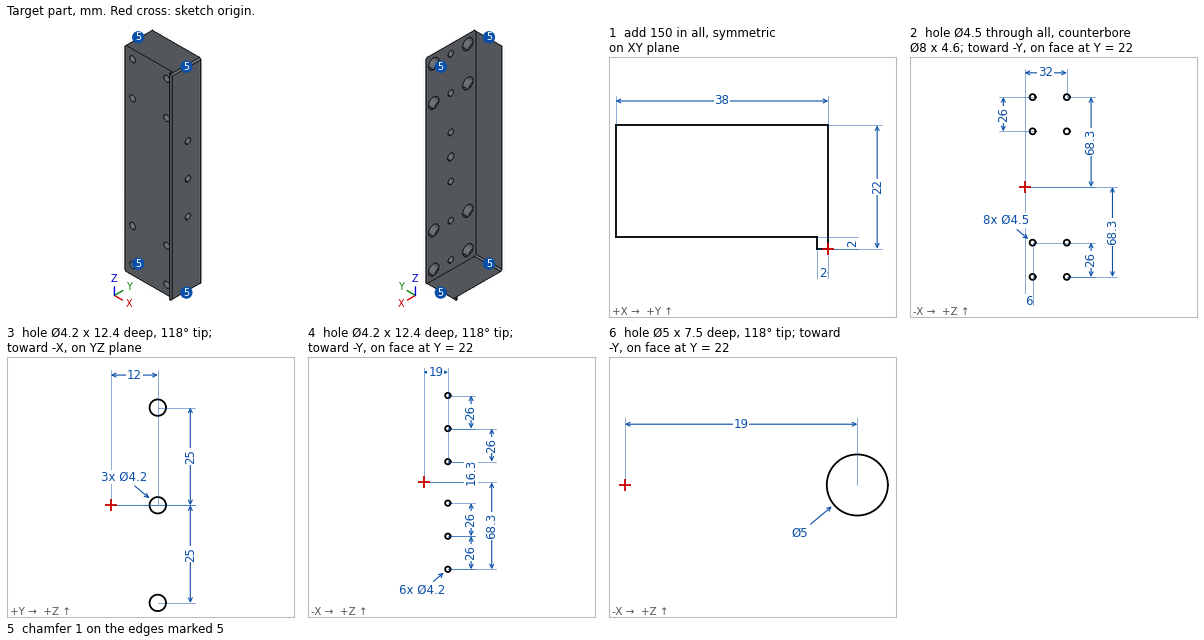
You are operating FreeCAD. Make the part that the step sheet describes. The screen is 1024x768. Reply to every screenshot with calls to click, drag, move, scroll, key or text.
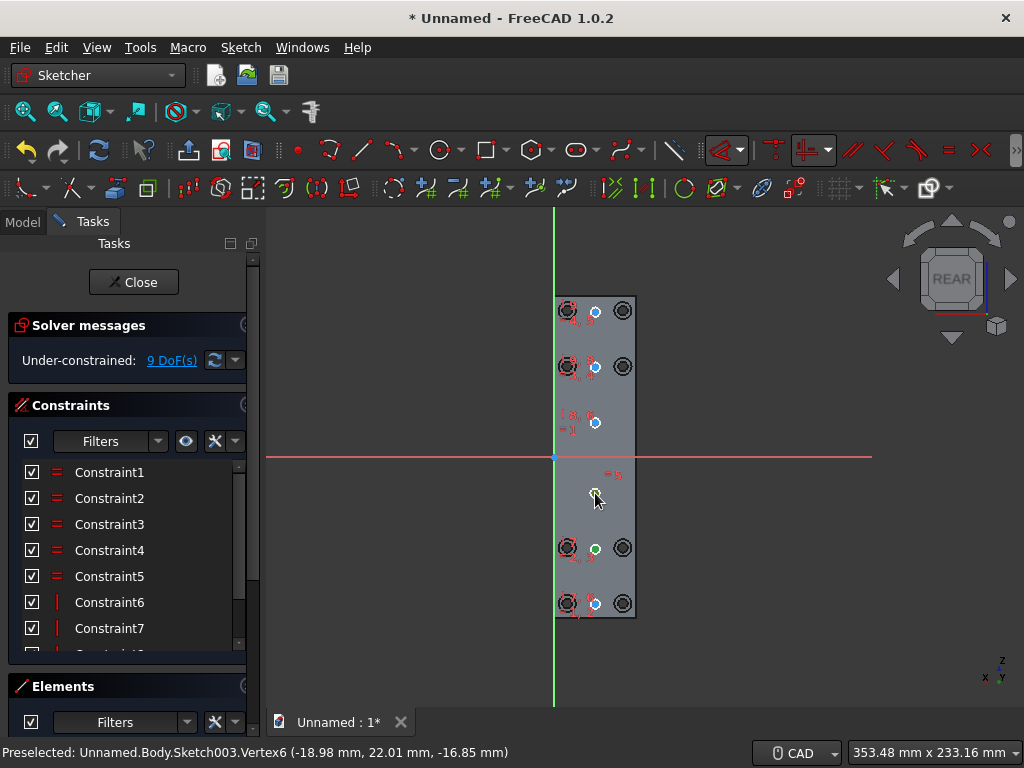
key(v)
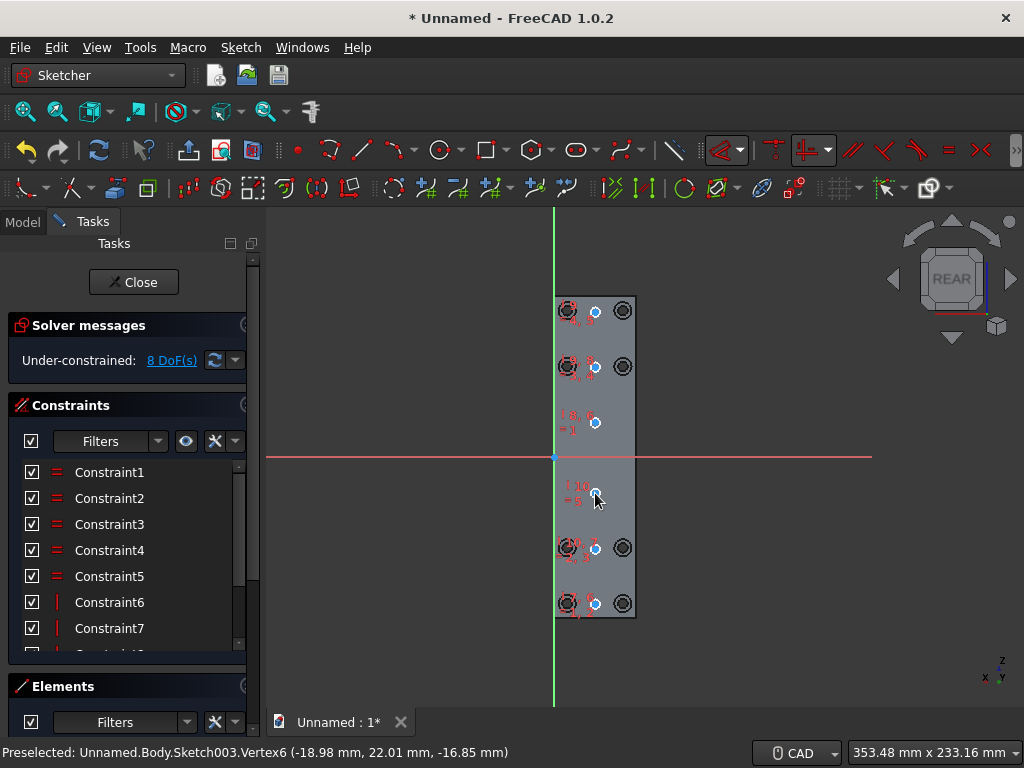
scroll(596, 418, up, 8)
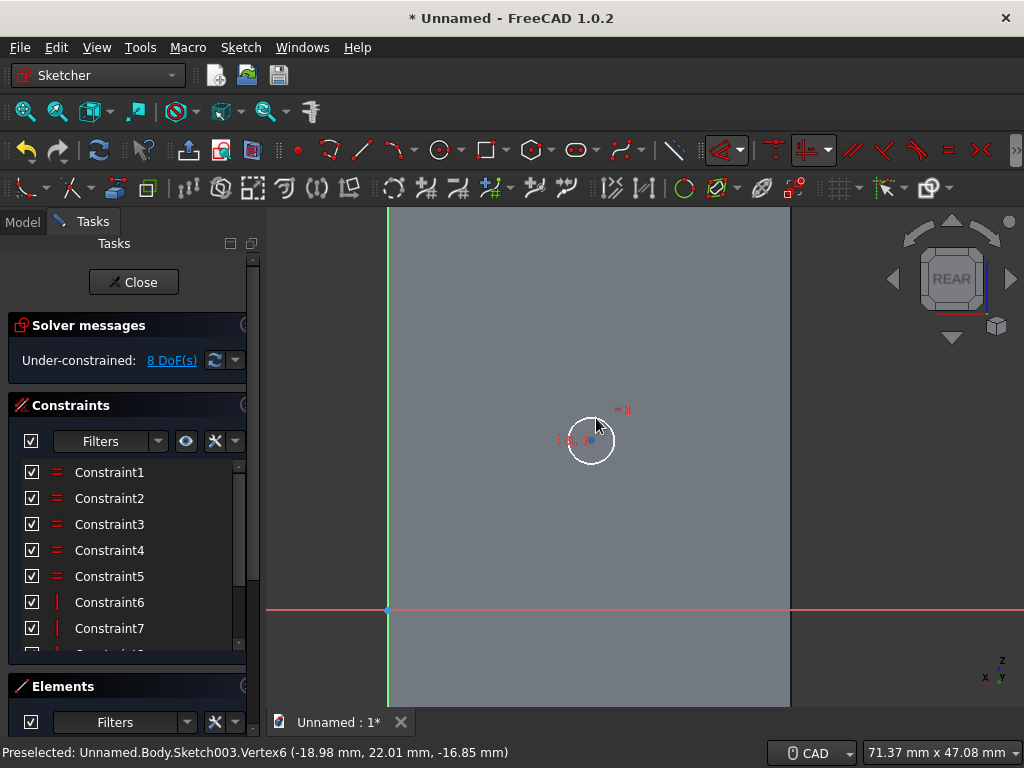
click(592, 418)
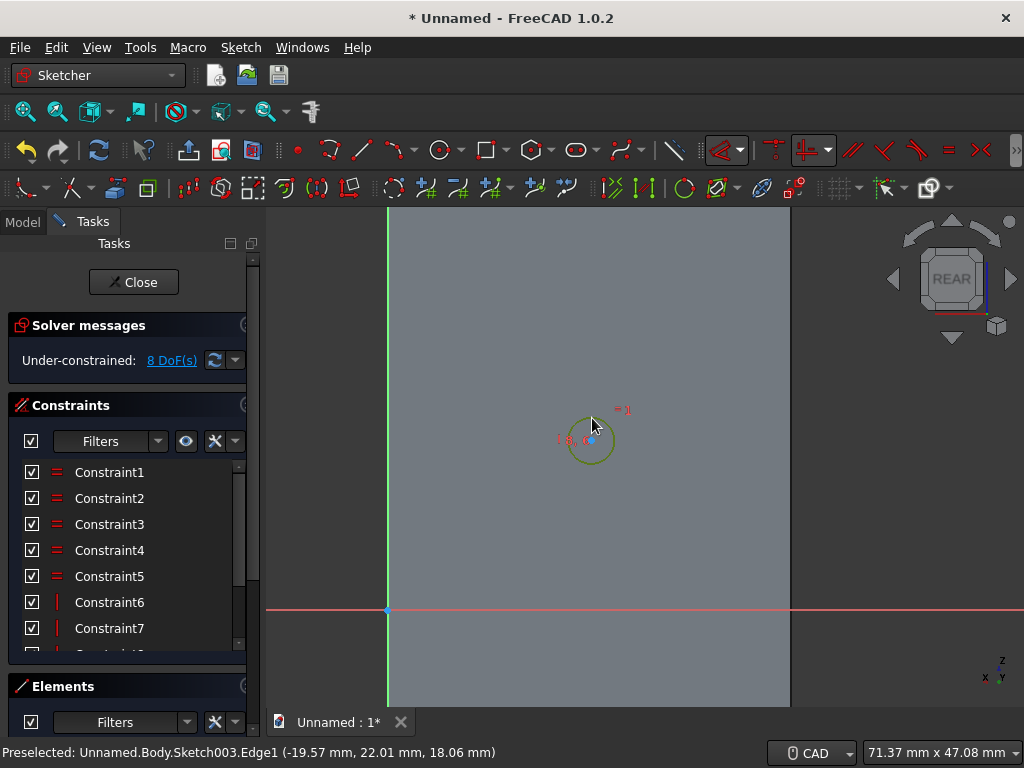
key(k)
key(o)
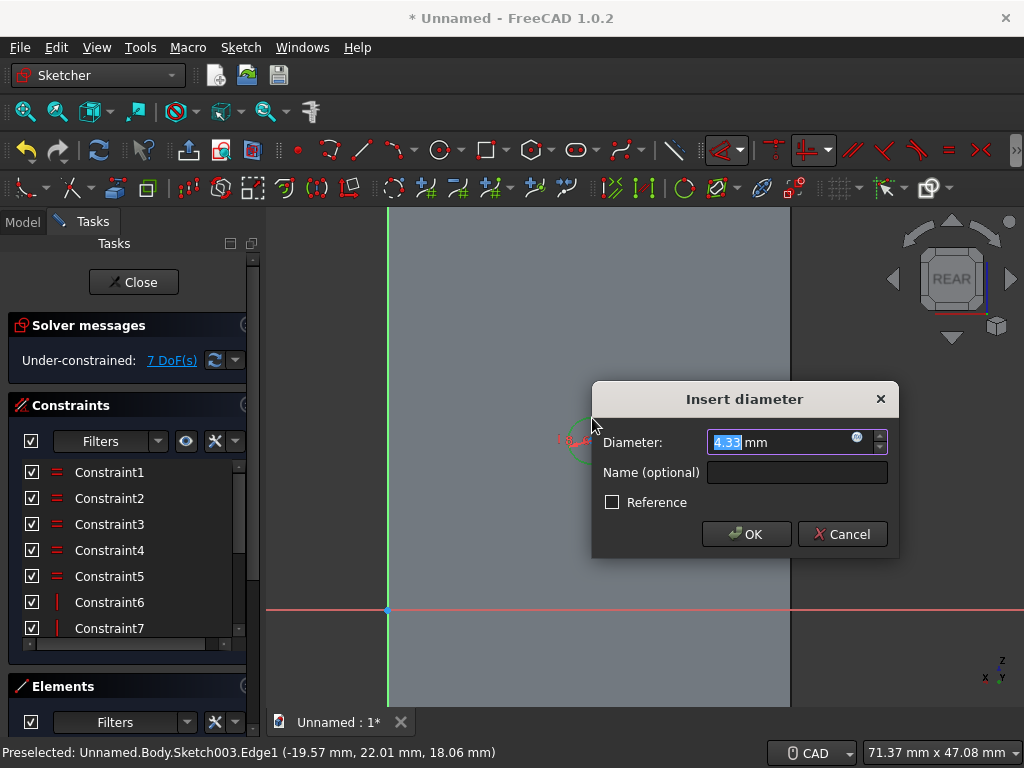
text(4.2)
key(Return)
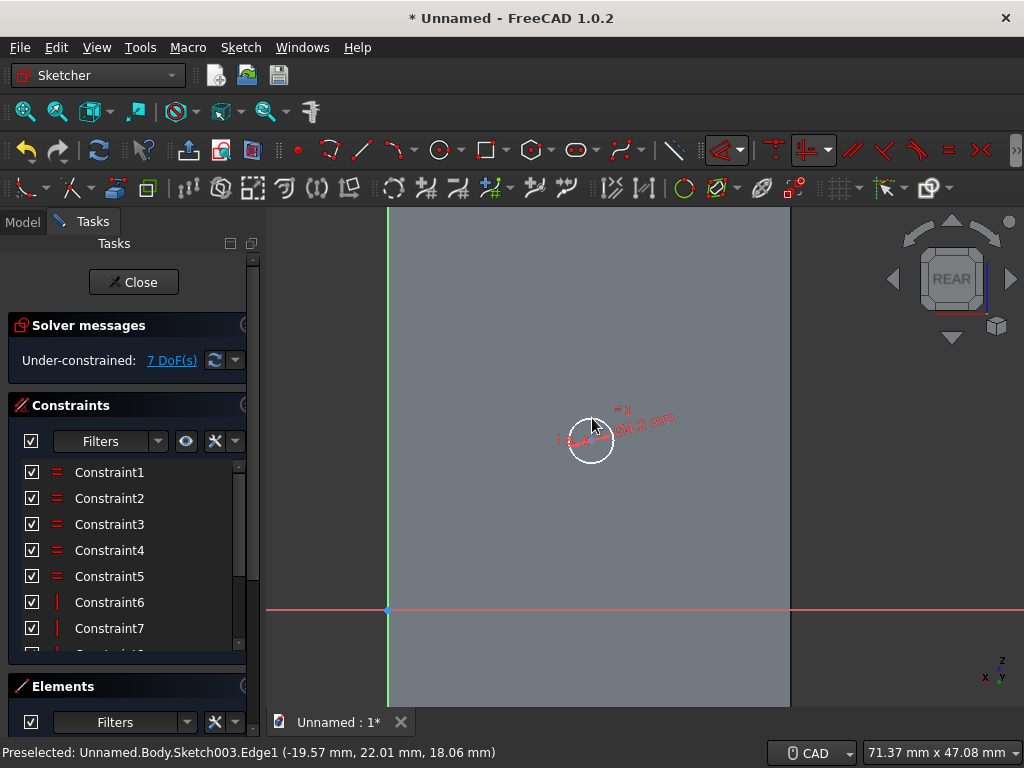
scroll(596, 418, down, 8)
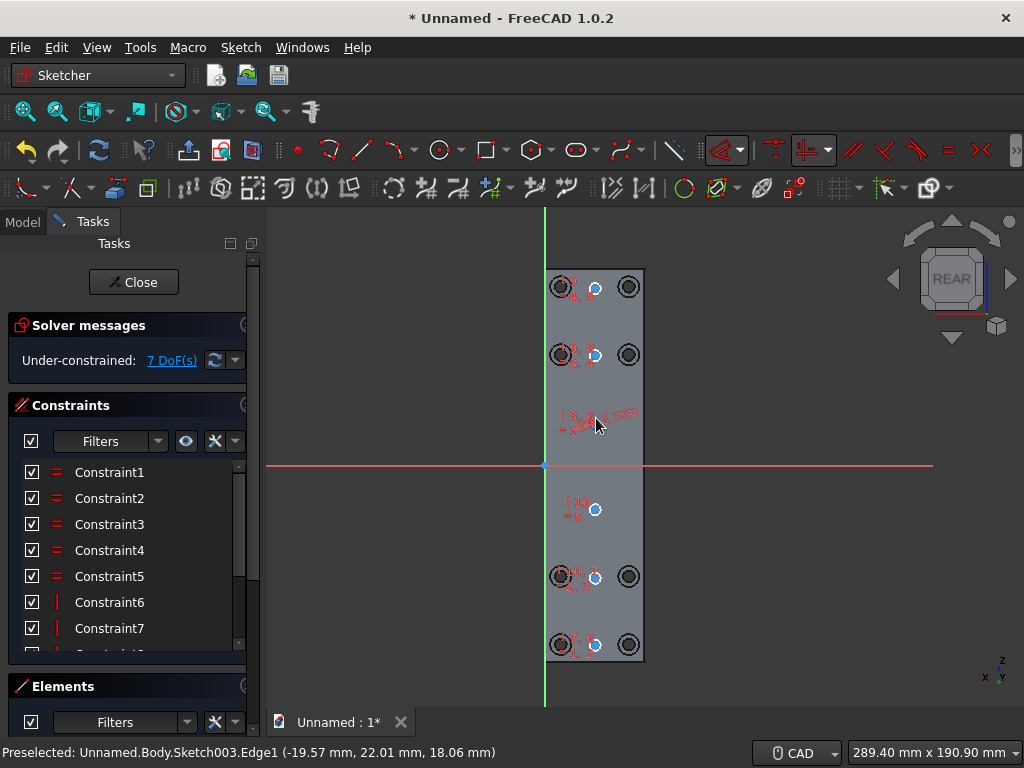
click(595, 423)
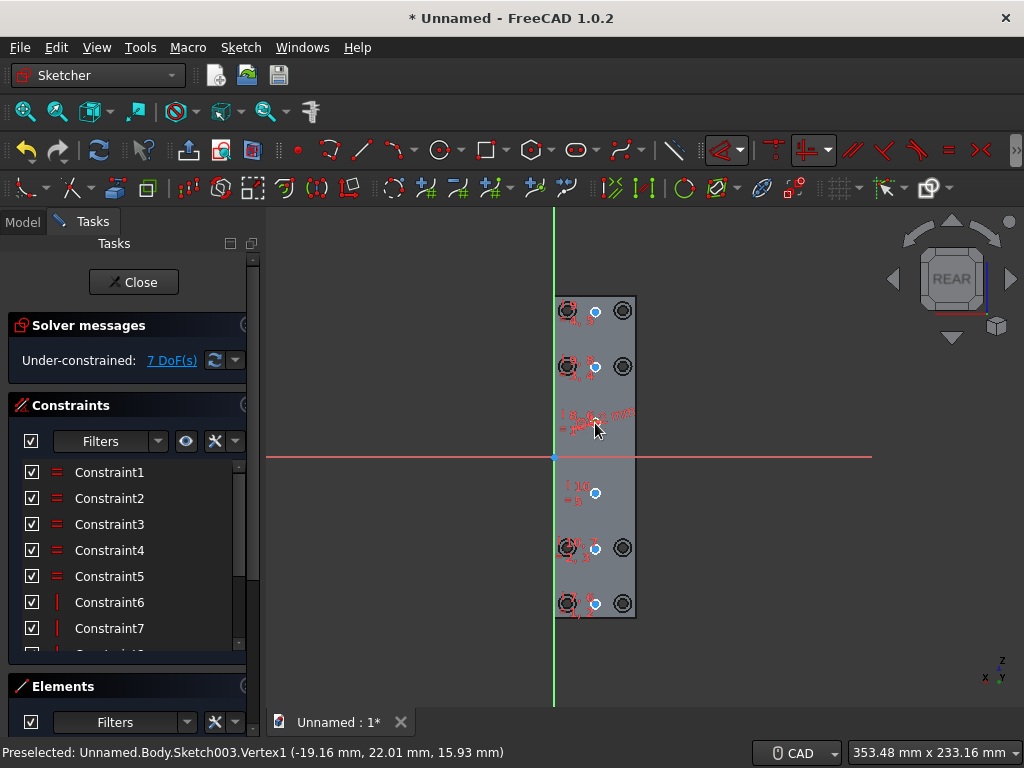
key(l)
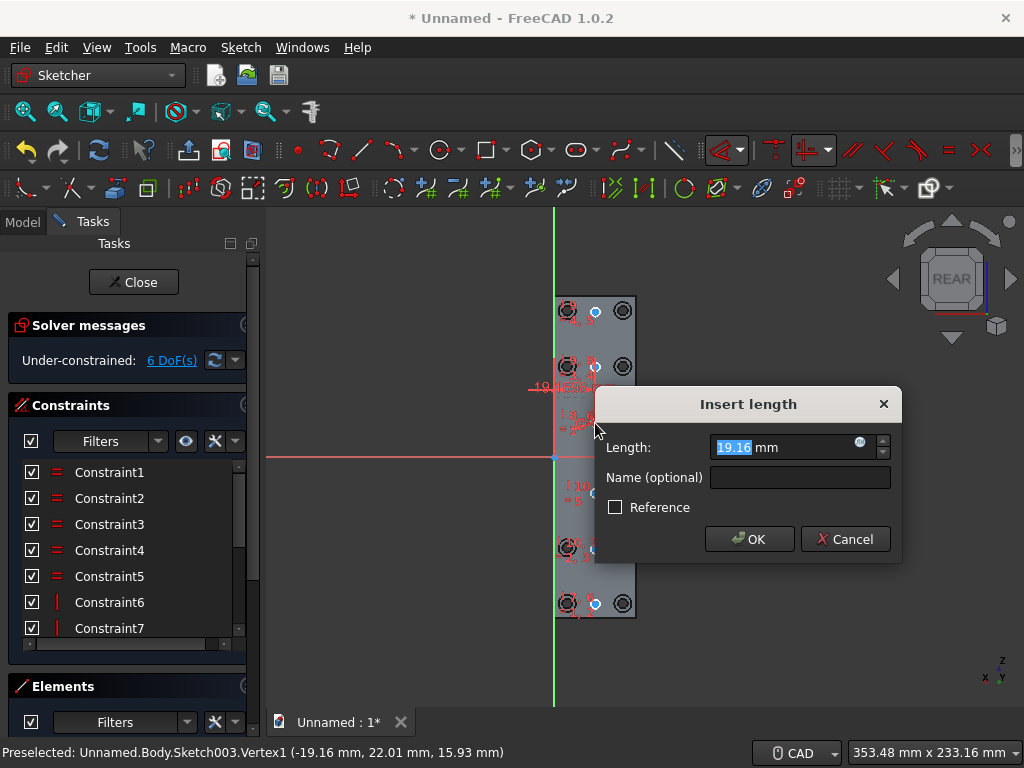
text(19)
key(Return)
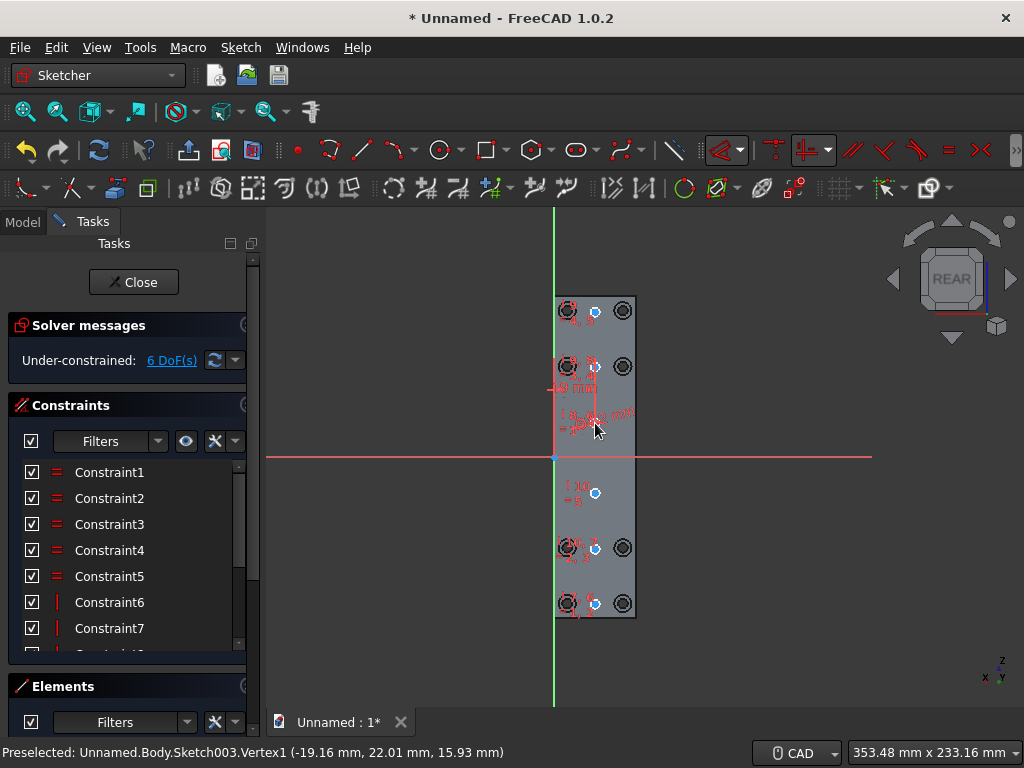
click(595, 604)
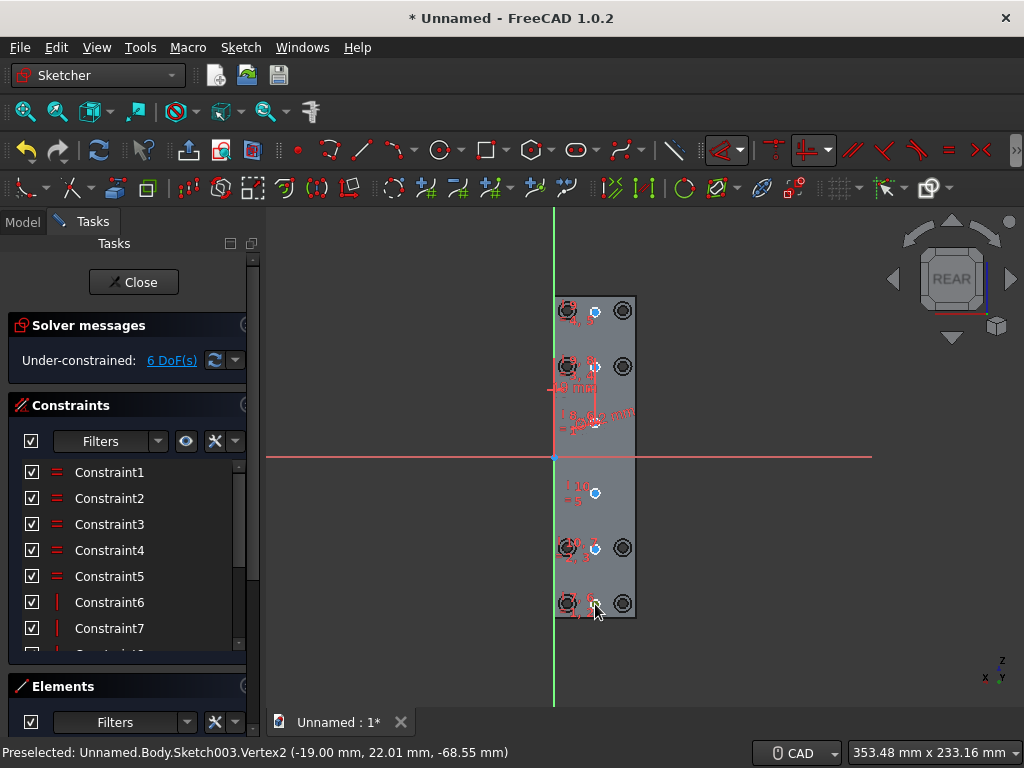
click(595, 549)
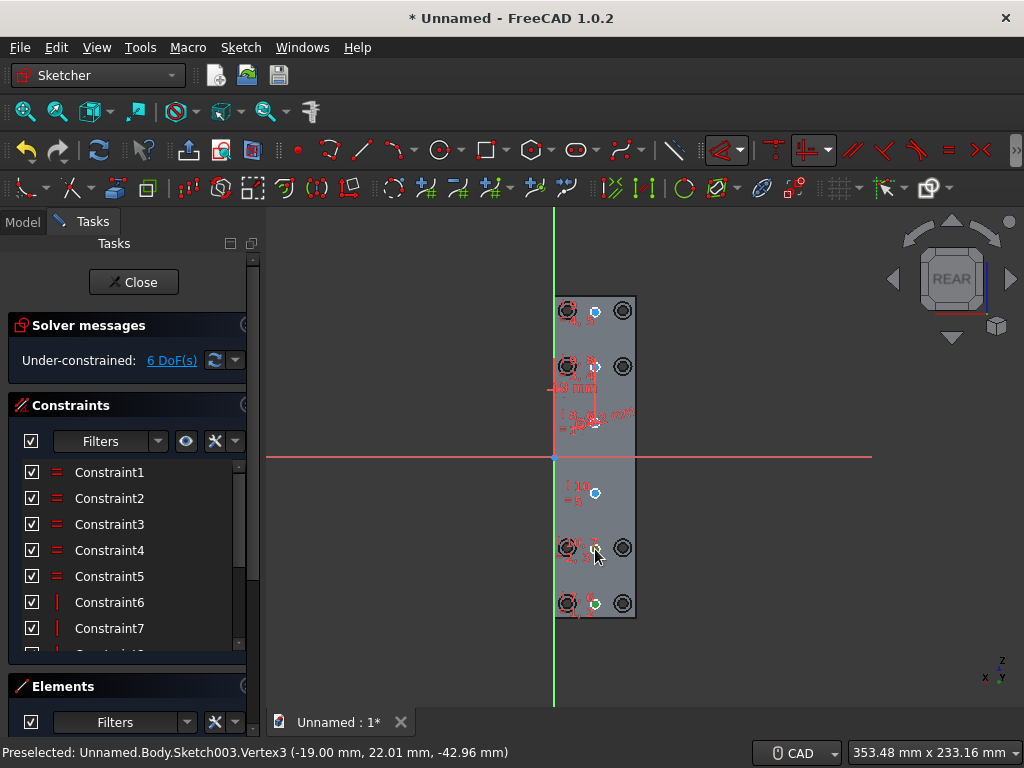
key(i)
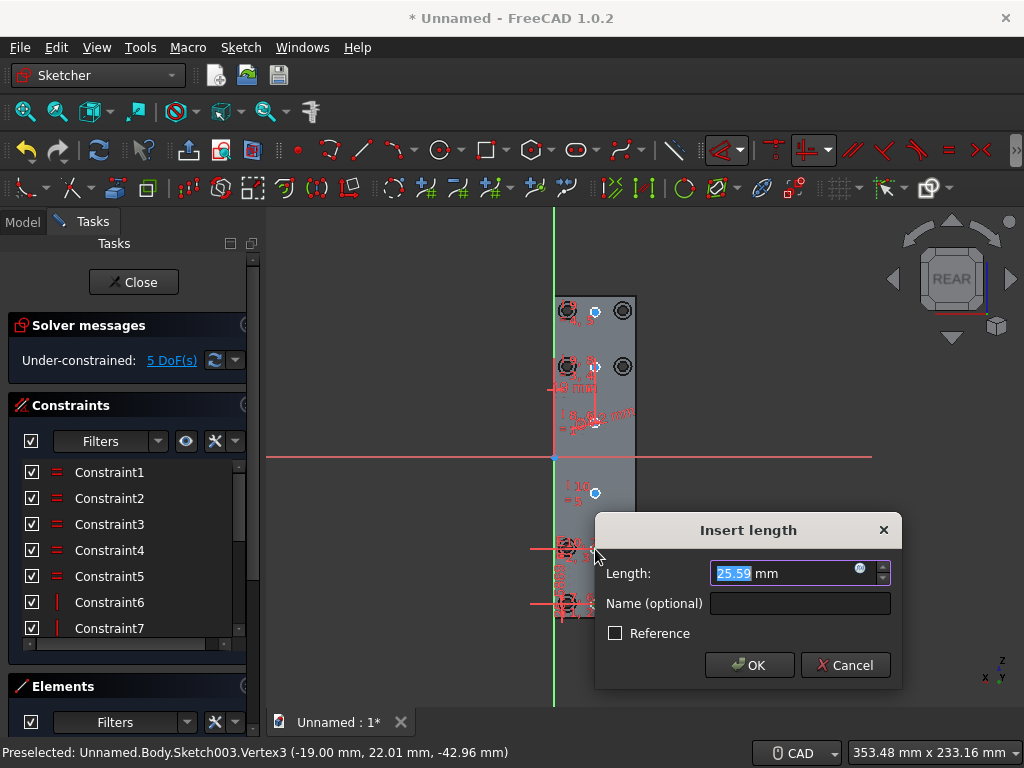
text(26)
key(Return)